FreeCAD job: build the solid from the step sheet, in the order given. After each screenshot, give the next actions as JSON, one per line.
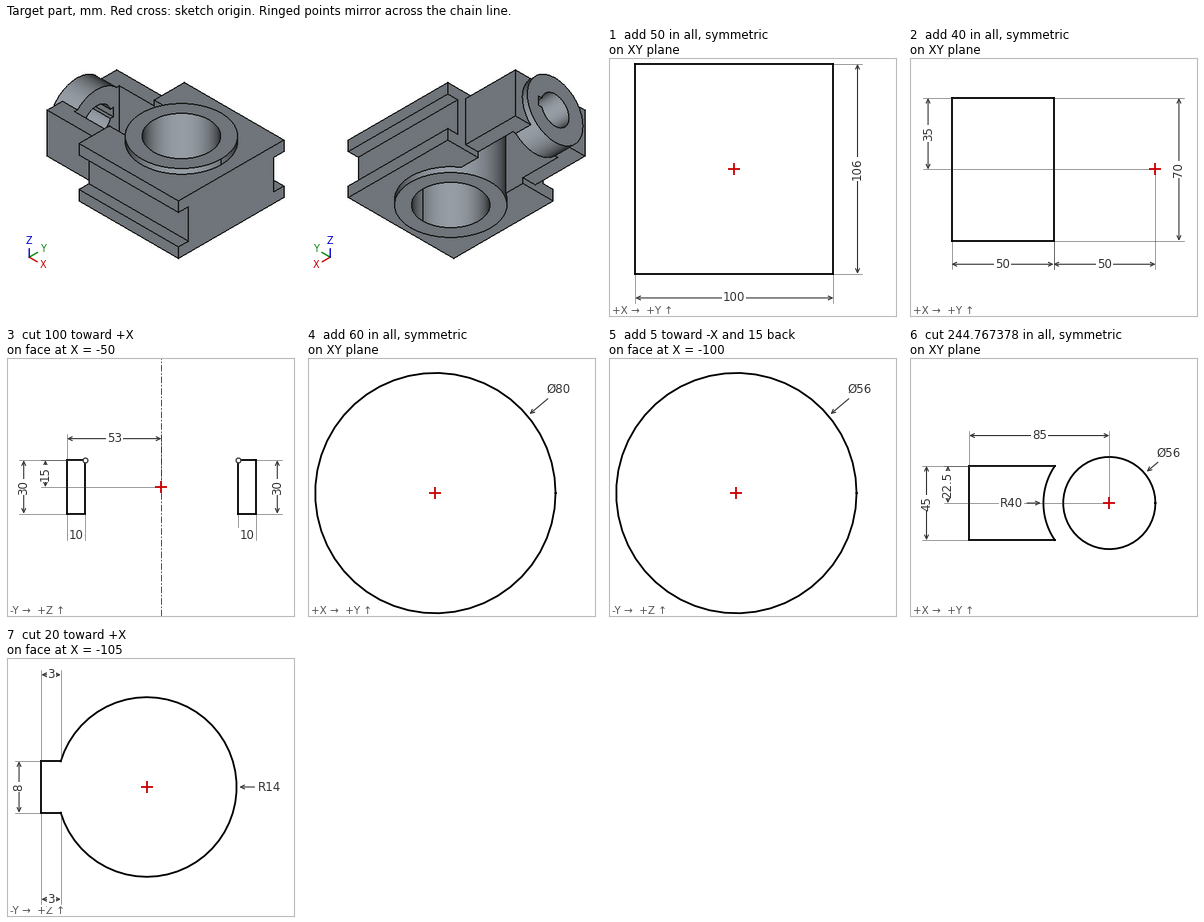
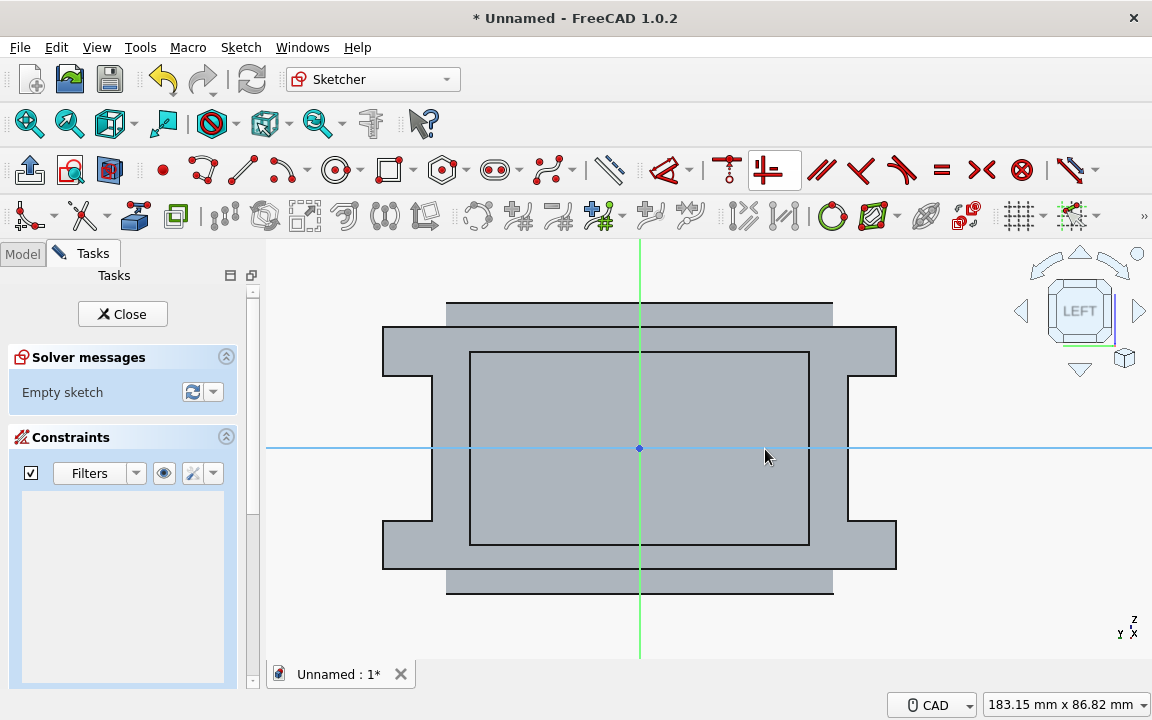
{"action": "left_click", "coordinate": [336, 170]}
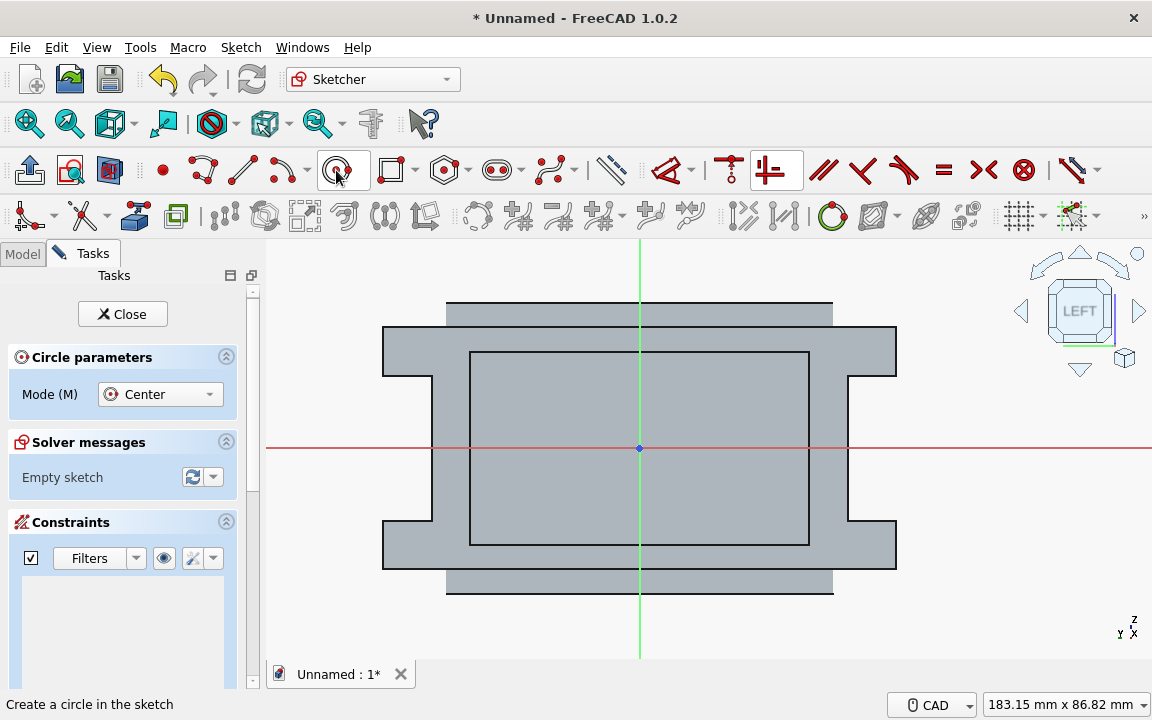
{"action": "left_click", "coordinate": [640, 448]}
{"action": "mouse_move", "coordinate": [735, 353]}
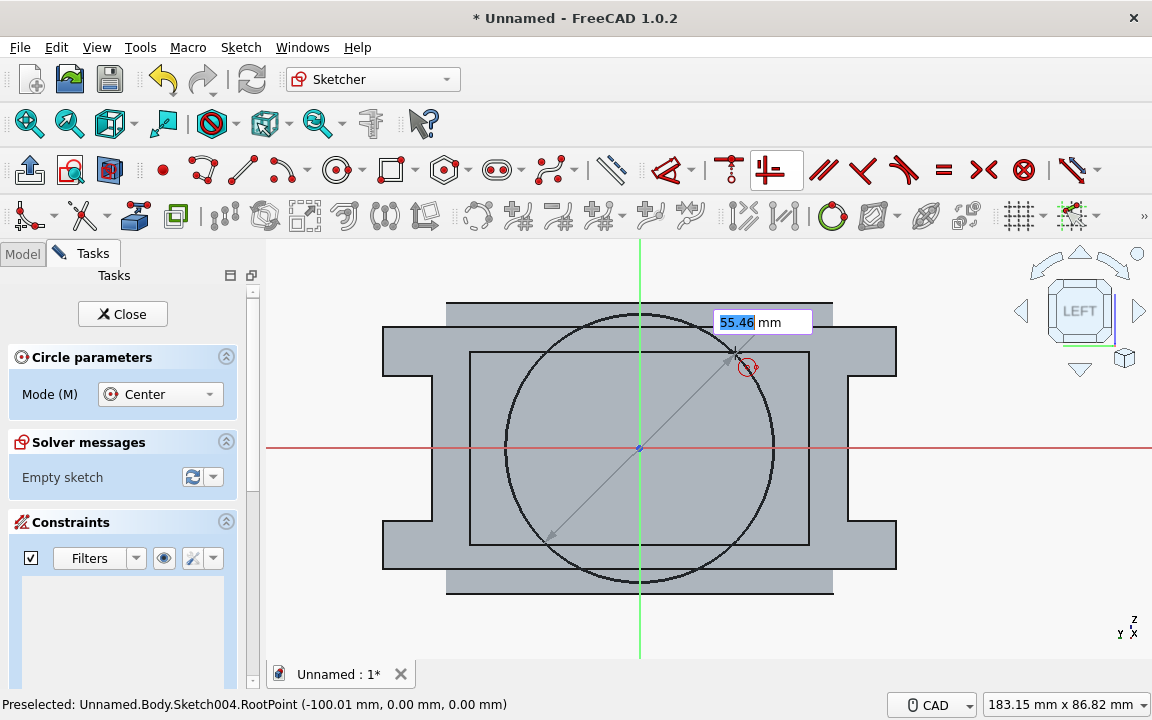
{"action": "type", "text": "56"}
{"action": "key", "text": "Return"}
{"action": "key", "text": "Escape"}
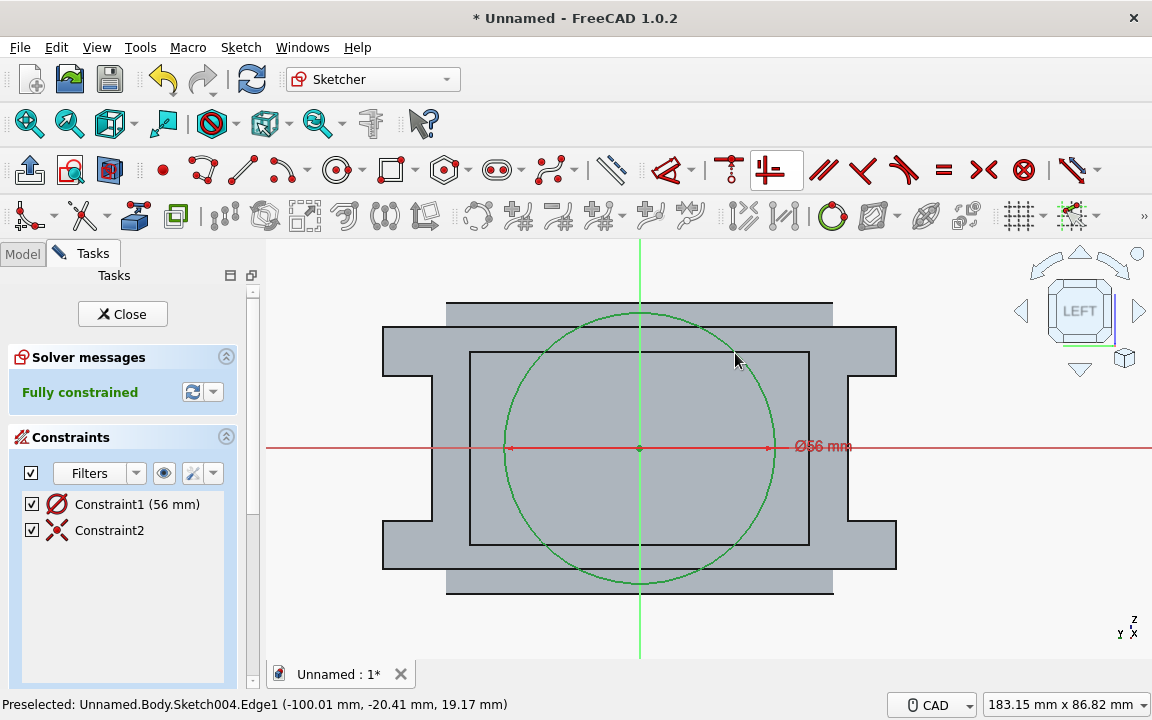
{"action": "left_click", "coordinate": [123, 314]}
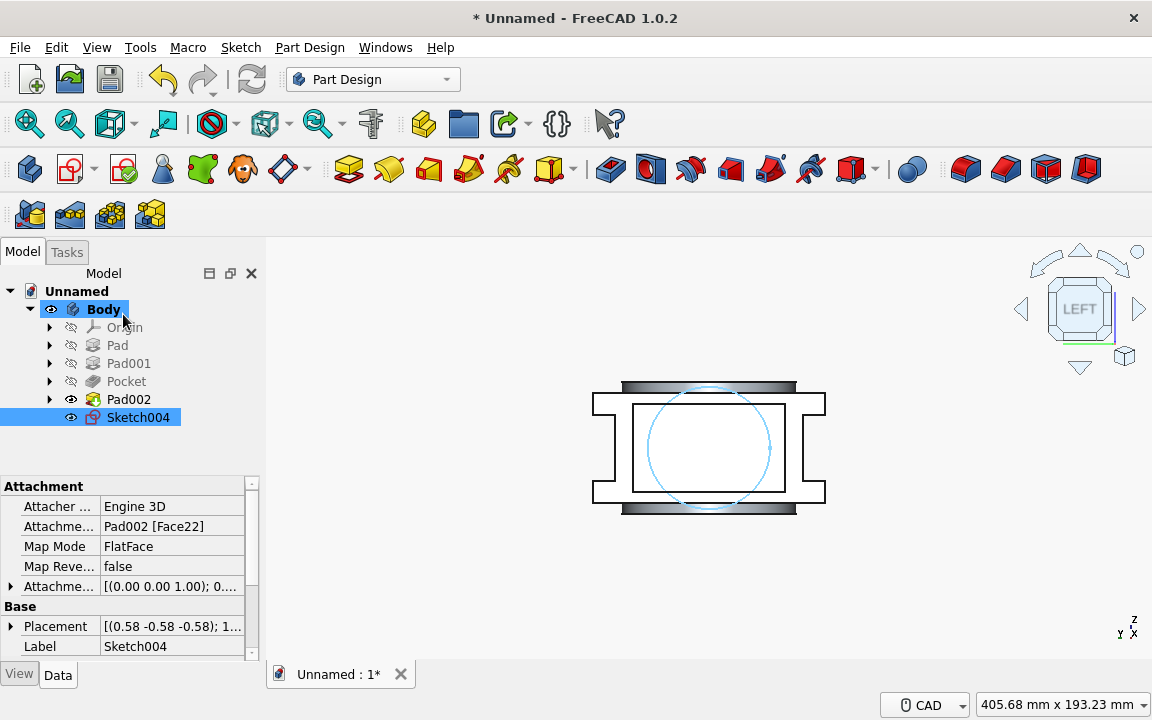
{"action": "left_click", "coordinate": [350, 170]}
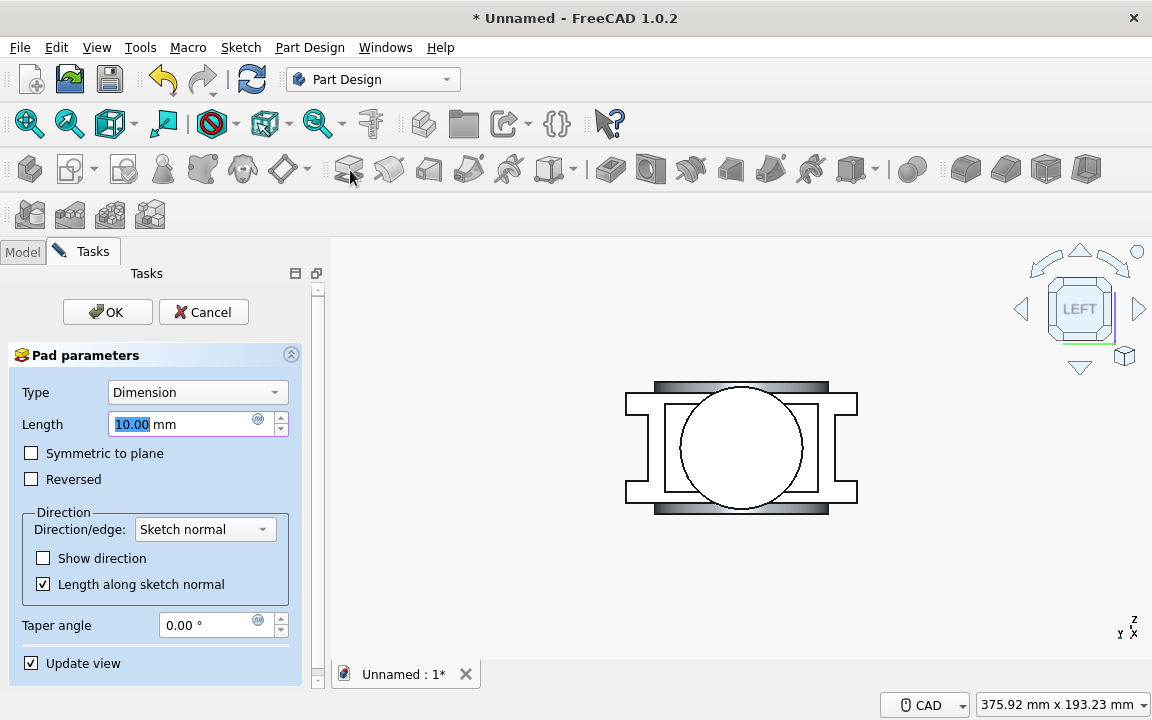
{"action": "left_click", "coordinate": [198, 392]}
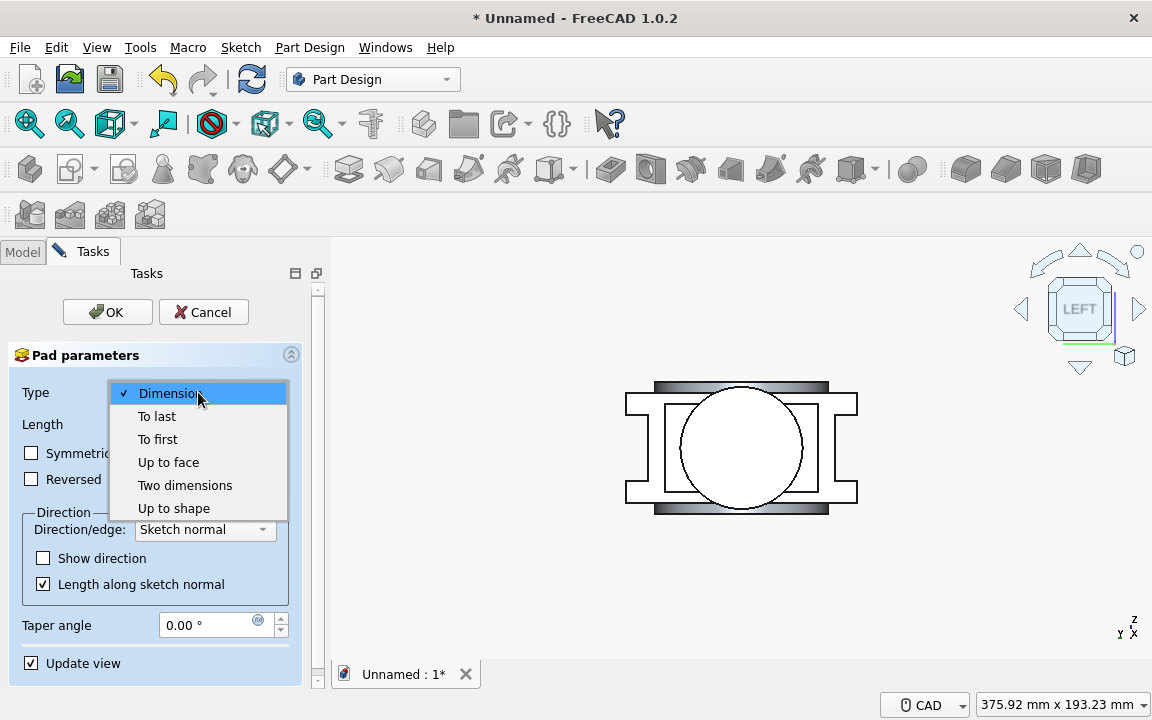
{"action": "left_click", "coordinate": [198, 486]}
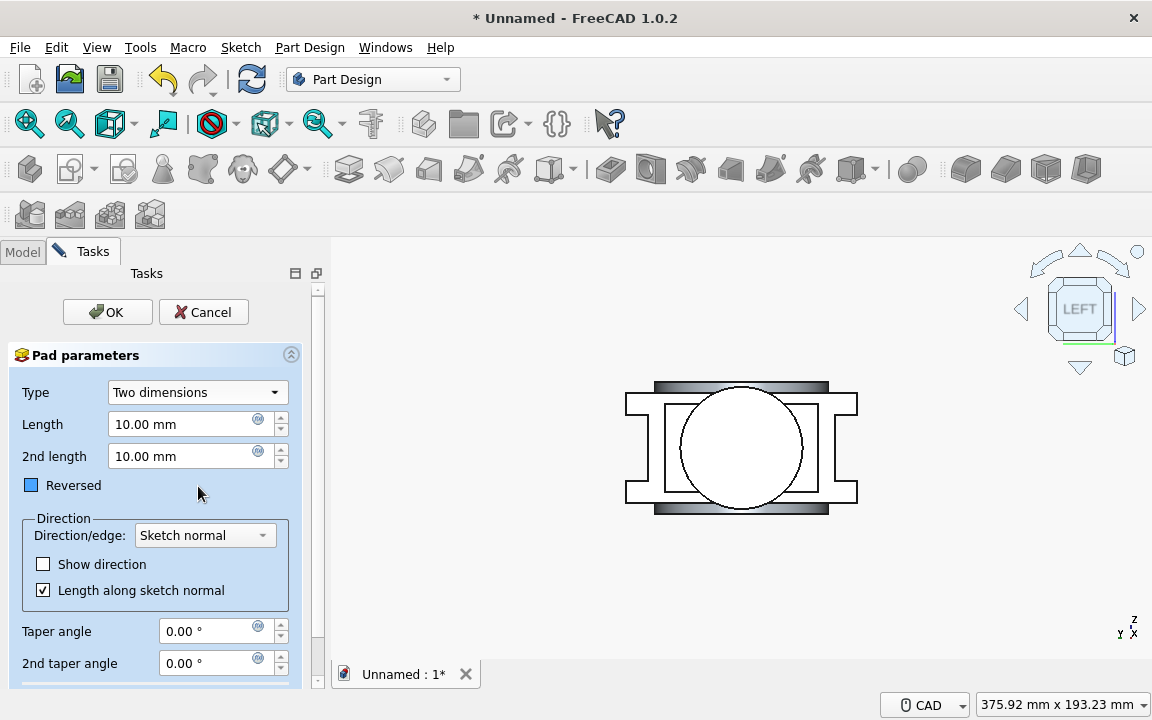
{"action": "triple_click", "coordinate": [190, 424]}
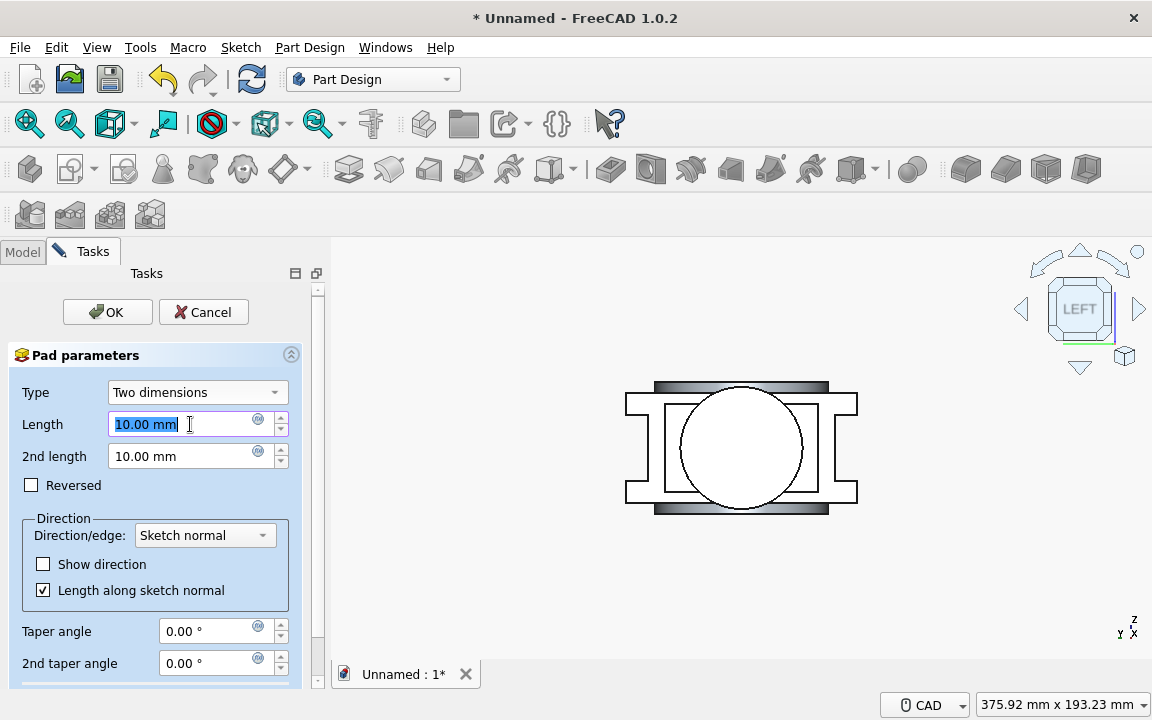
{"action": "type", "text": "5"}
{"action": "key", "text": "Tab"}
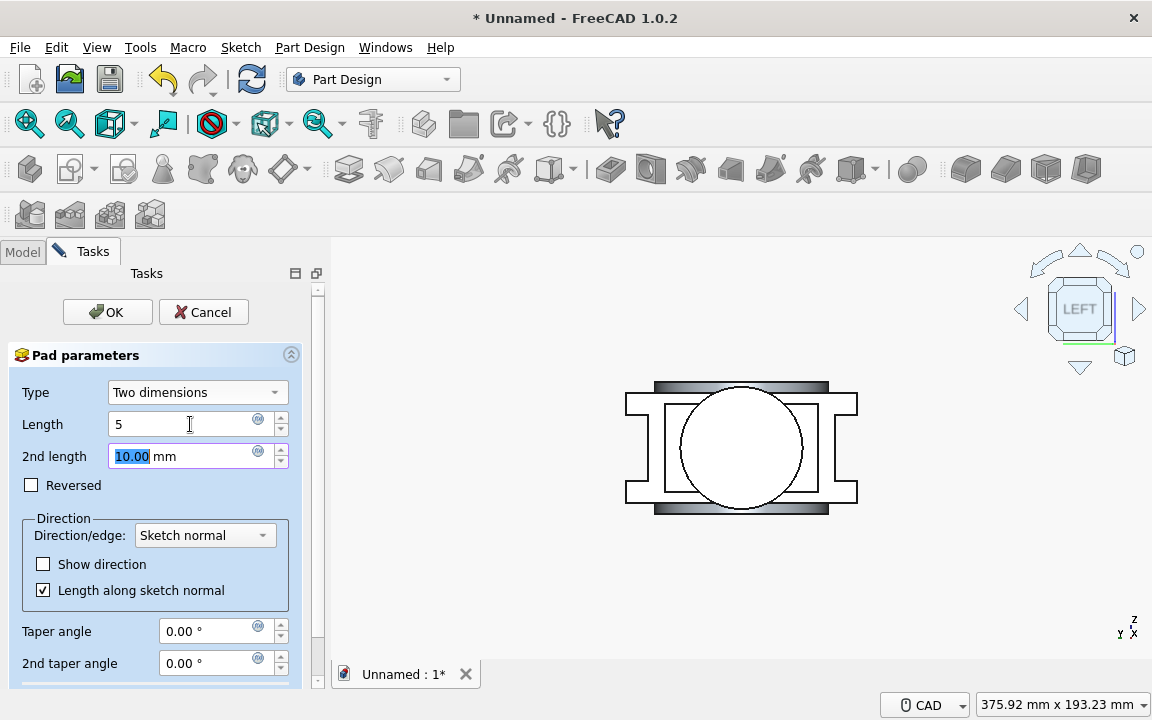
{"action": "type", "text": "15"}
{"action": "key", "text": "Tab"}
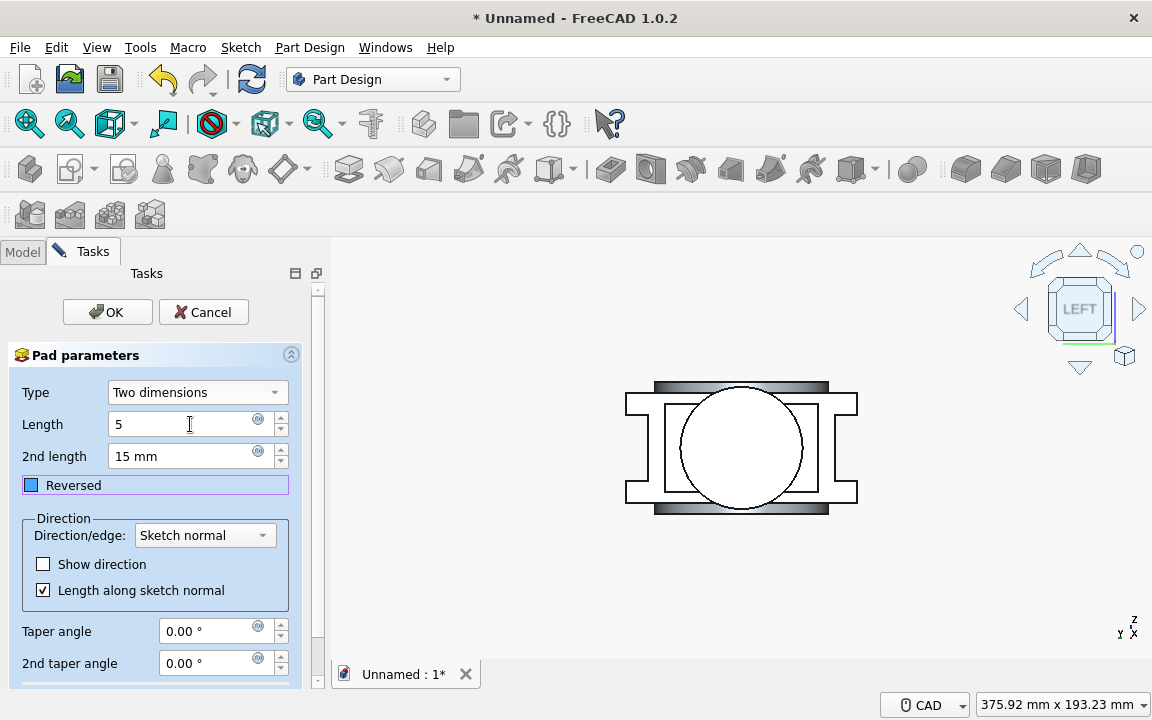
{"action": "left_click", "coordinate": [108, 312]}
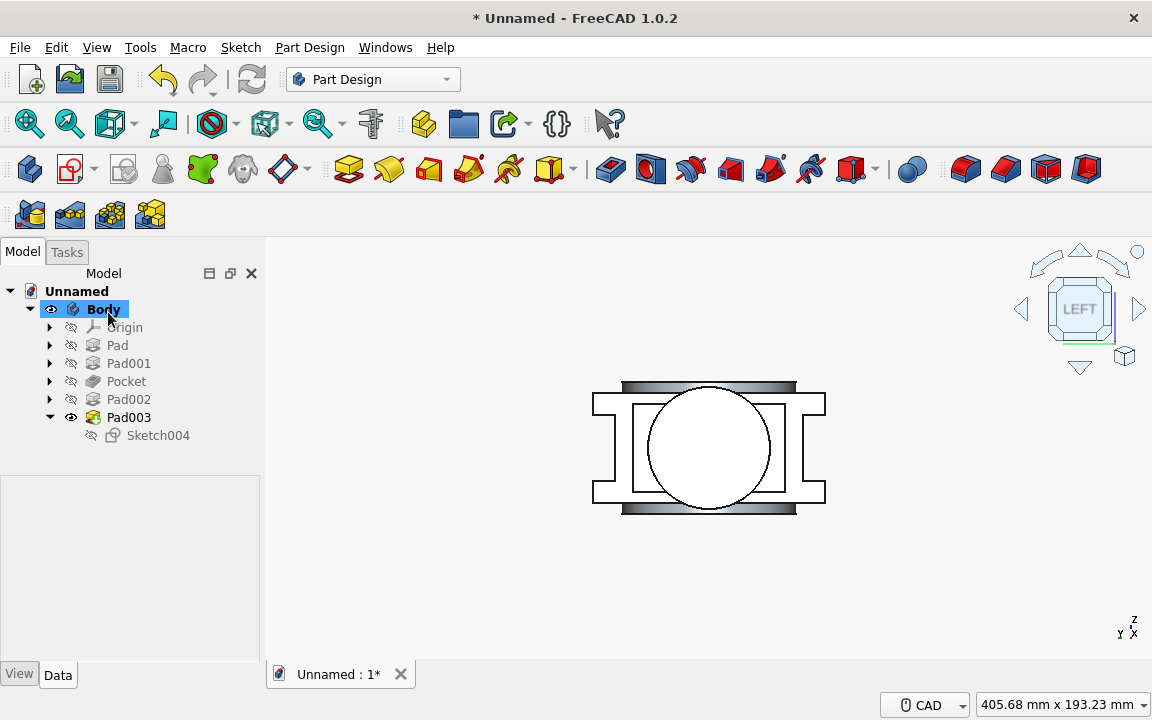
{"action": "left_click", "coordinate": [30, 124]}